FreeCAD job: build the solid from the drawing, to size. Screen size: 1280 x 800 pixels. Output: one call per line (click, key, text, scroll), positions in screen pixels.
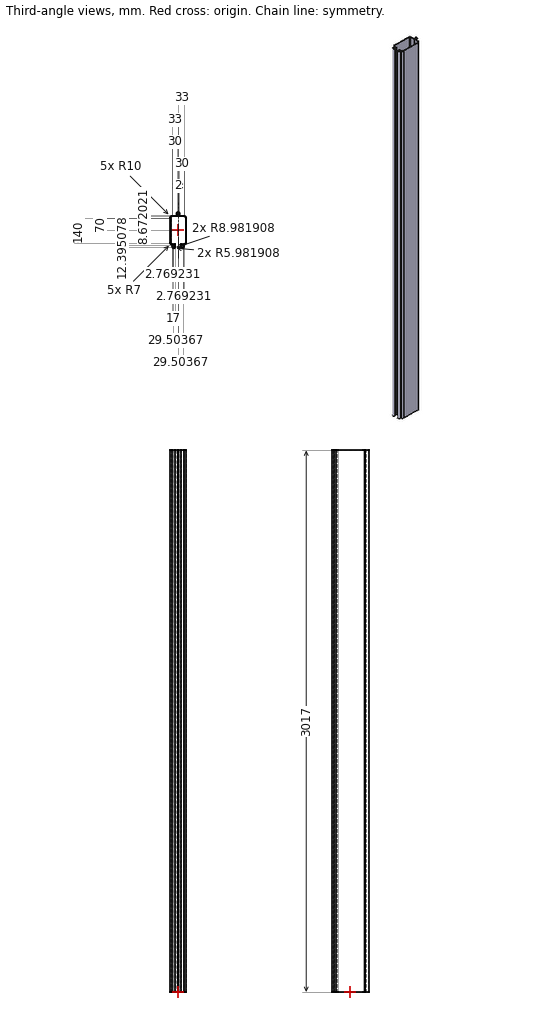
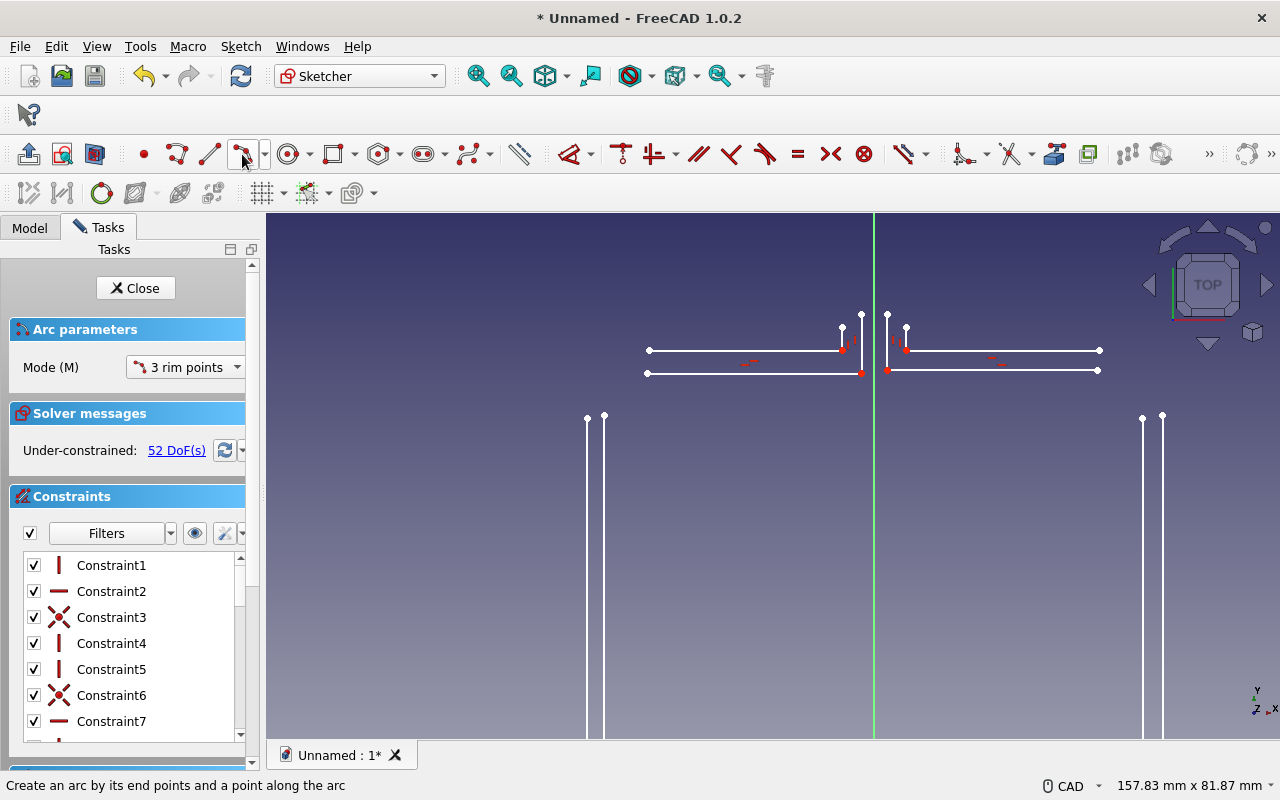
scroll(649, 350, down, 7)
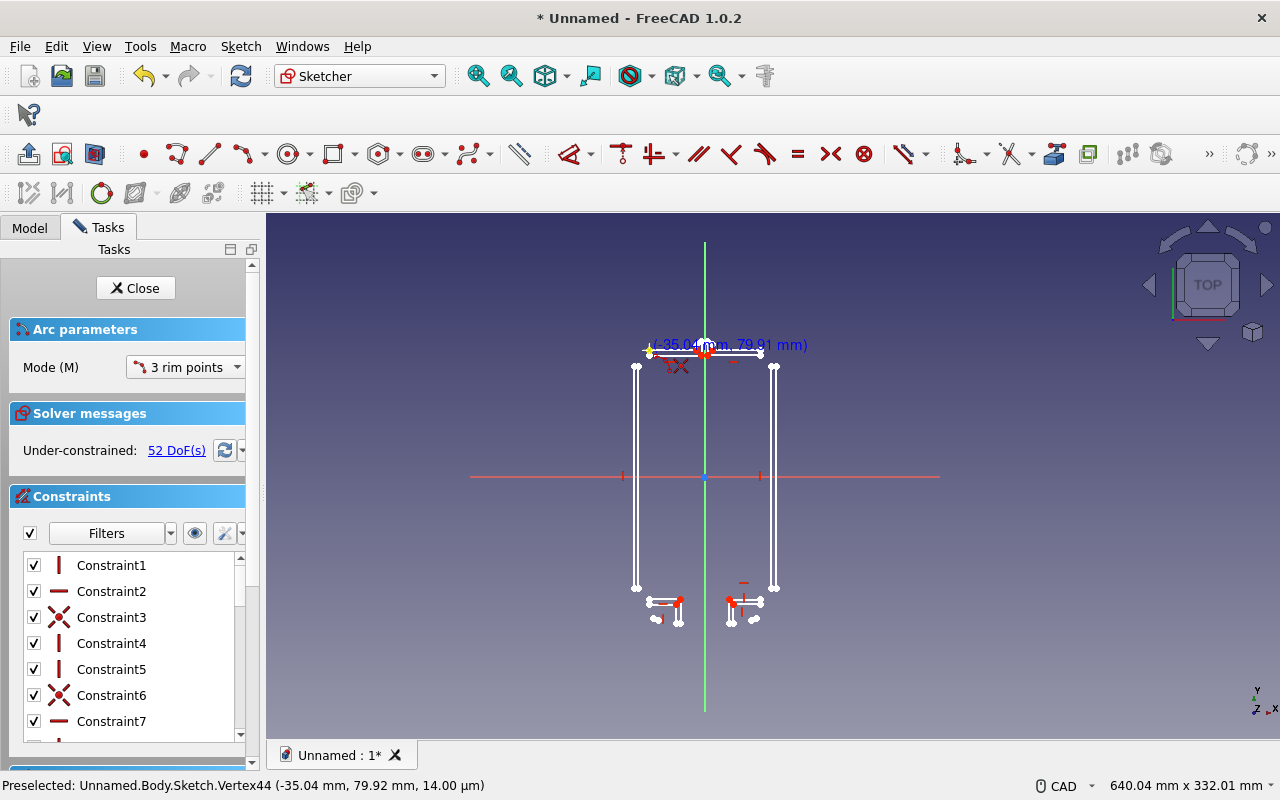
scroll(634, 588, up, 7)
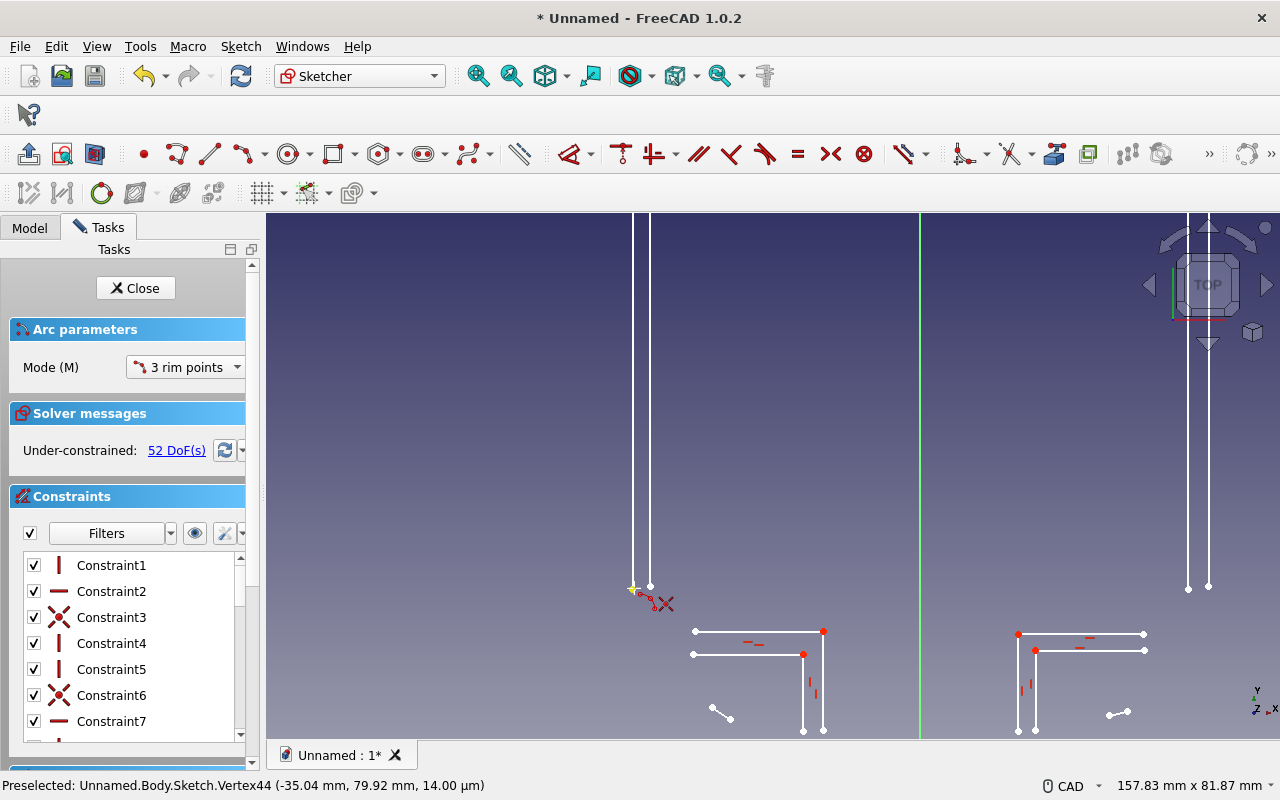
click(633, 590)
click(694, 655)
click(650, 631)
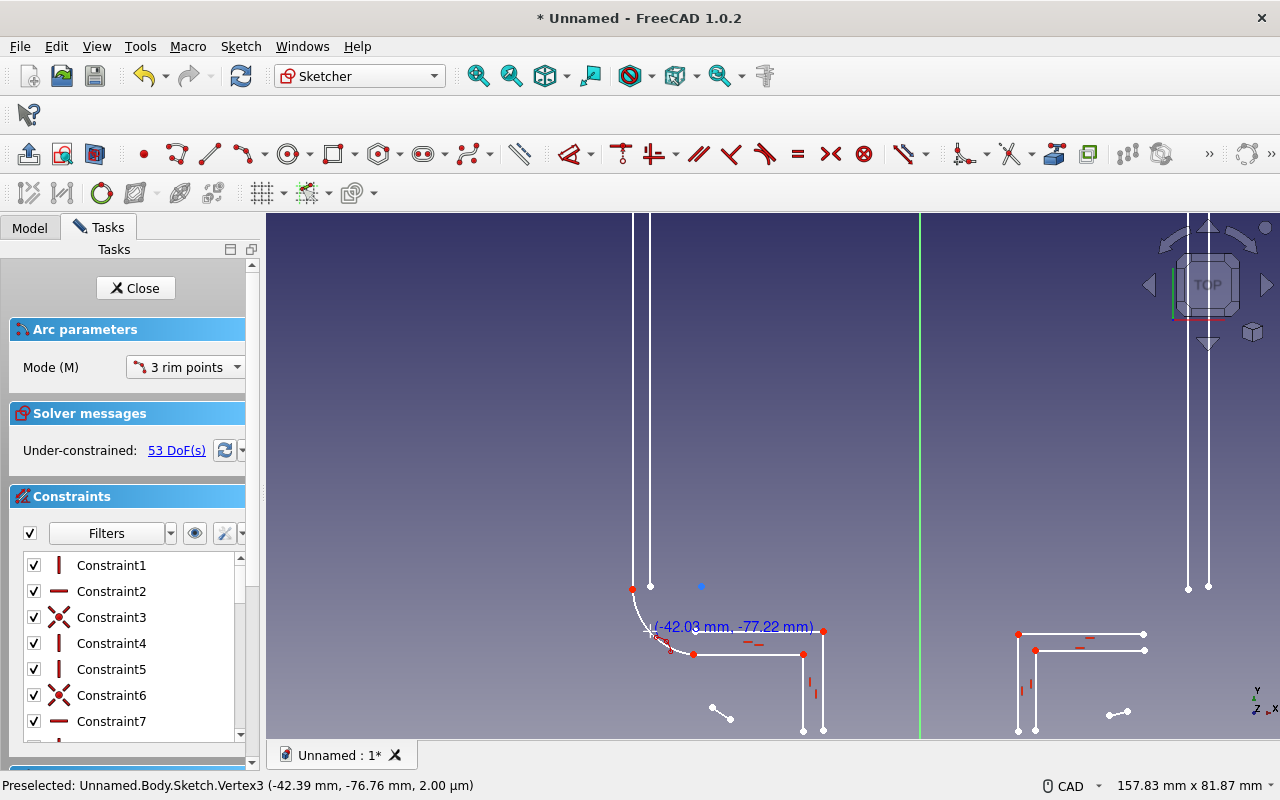
scroll(634, 589, down, 7)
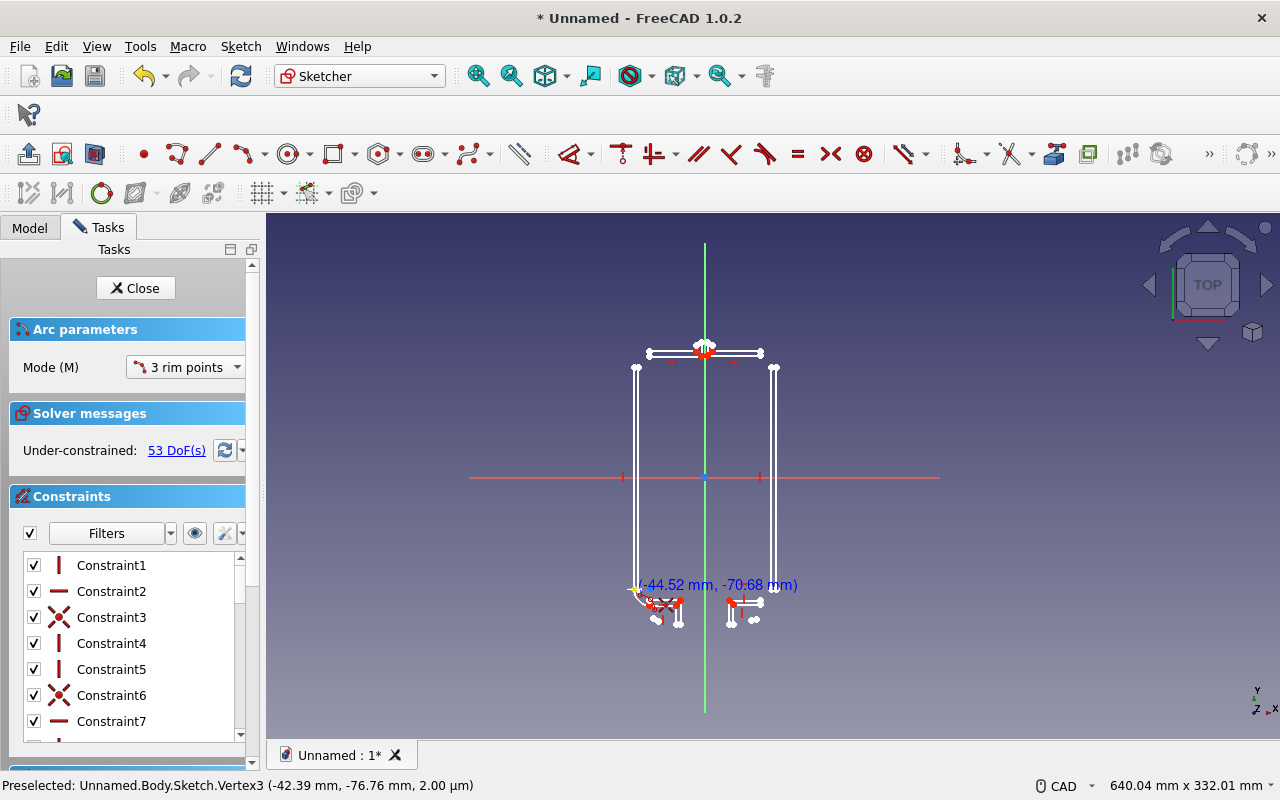
scroll(676, 624, up, 7)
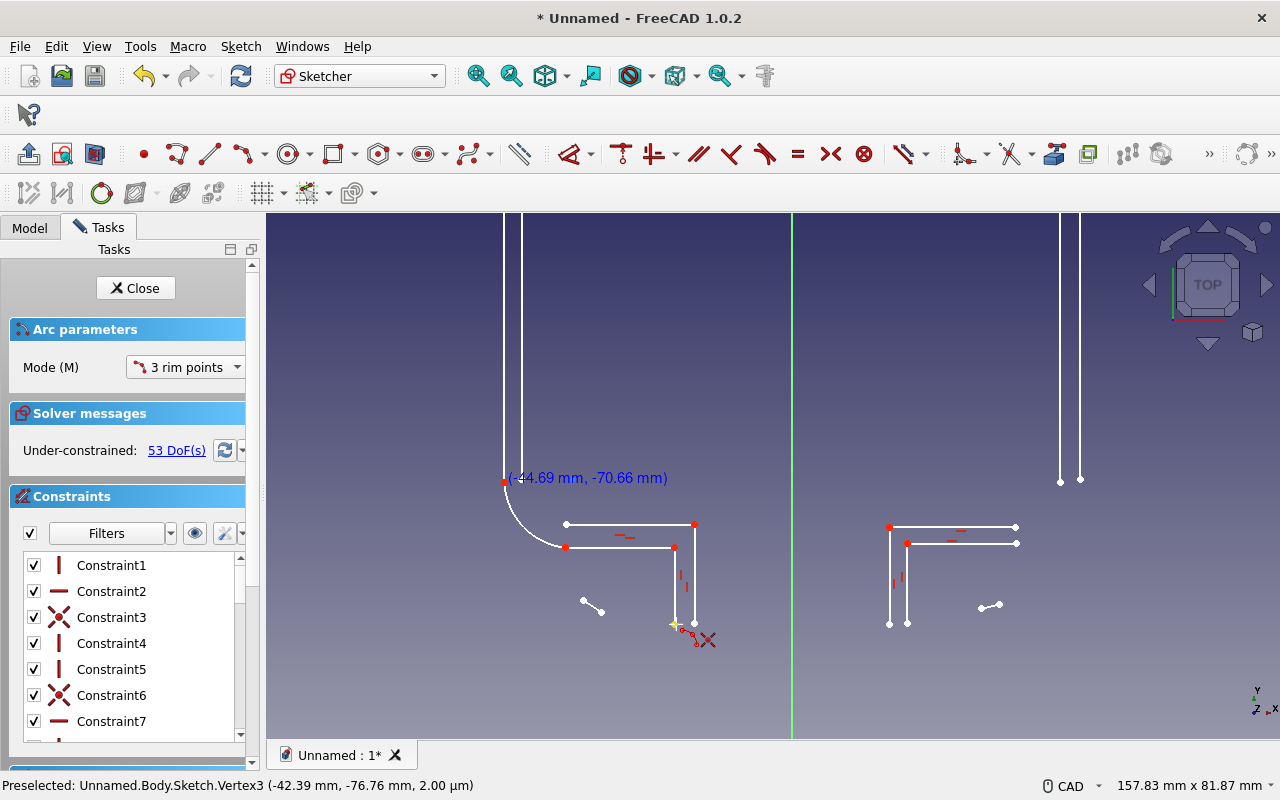
click(675, 625)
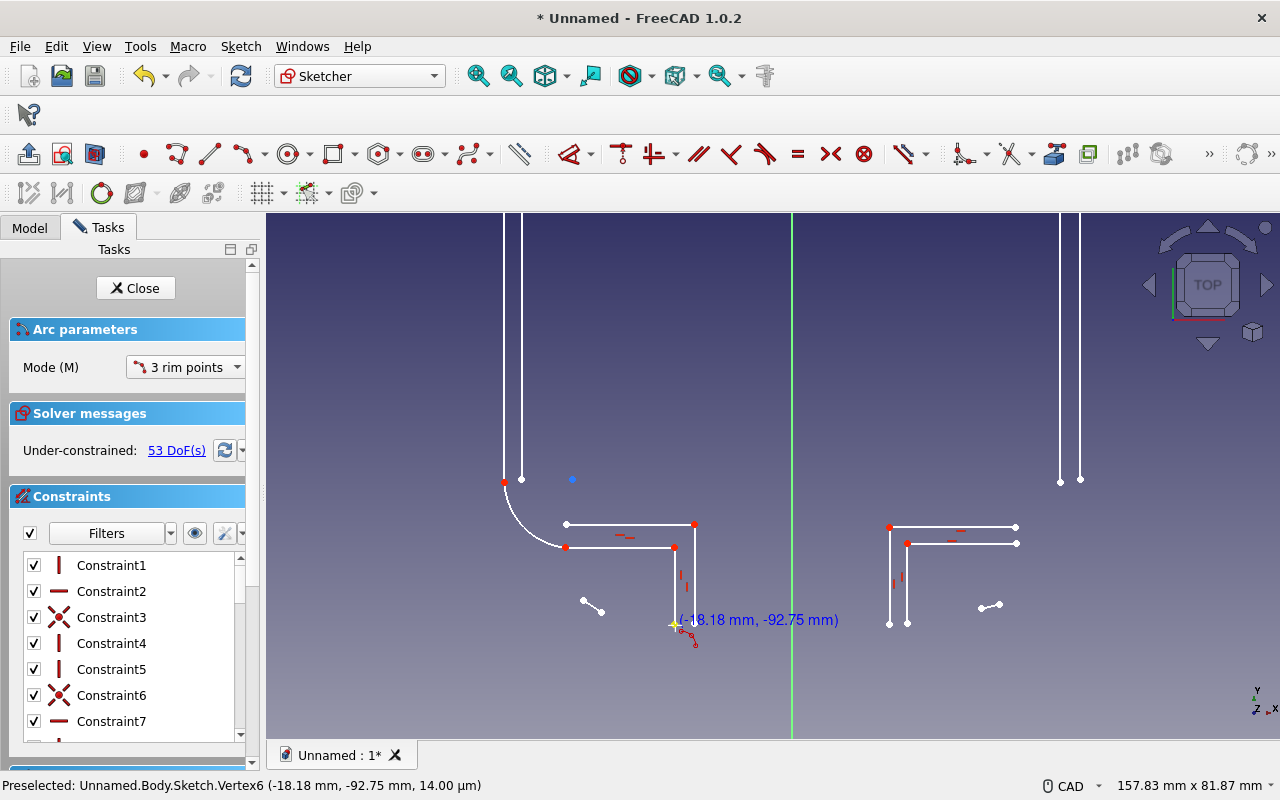
scroll(602, 608, up, 3)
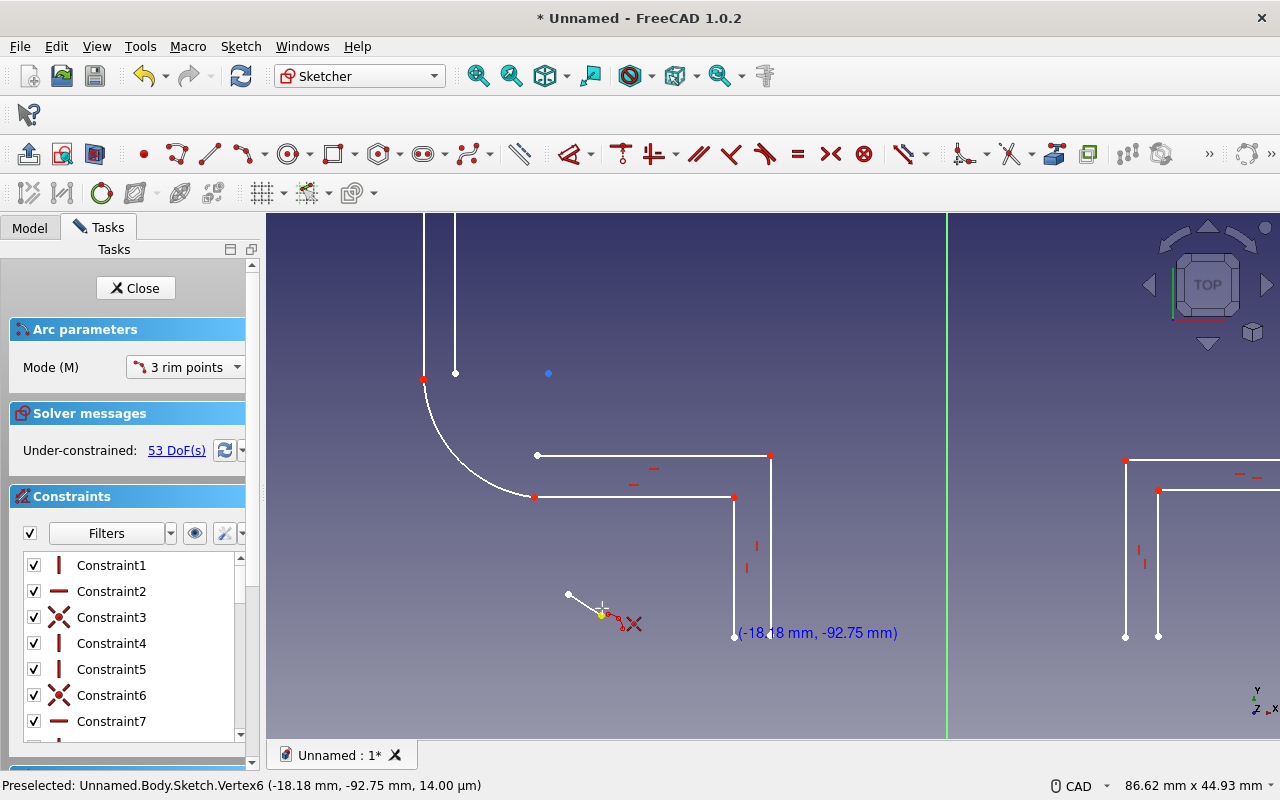
click(601, 616)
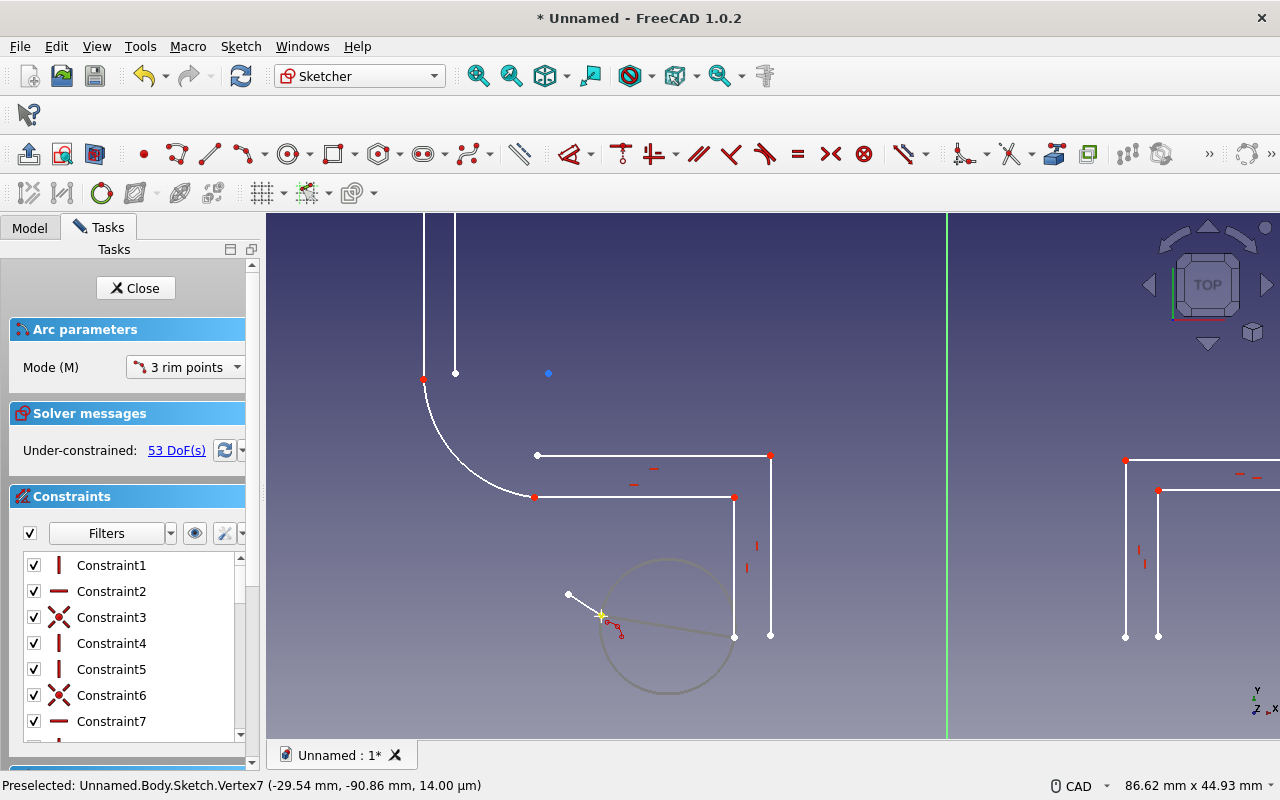
scroll(667, 622, down, 10)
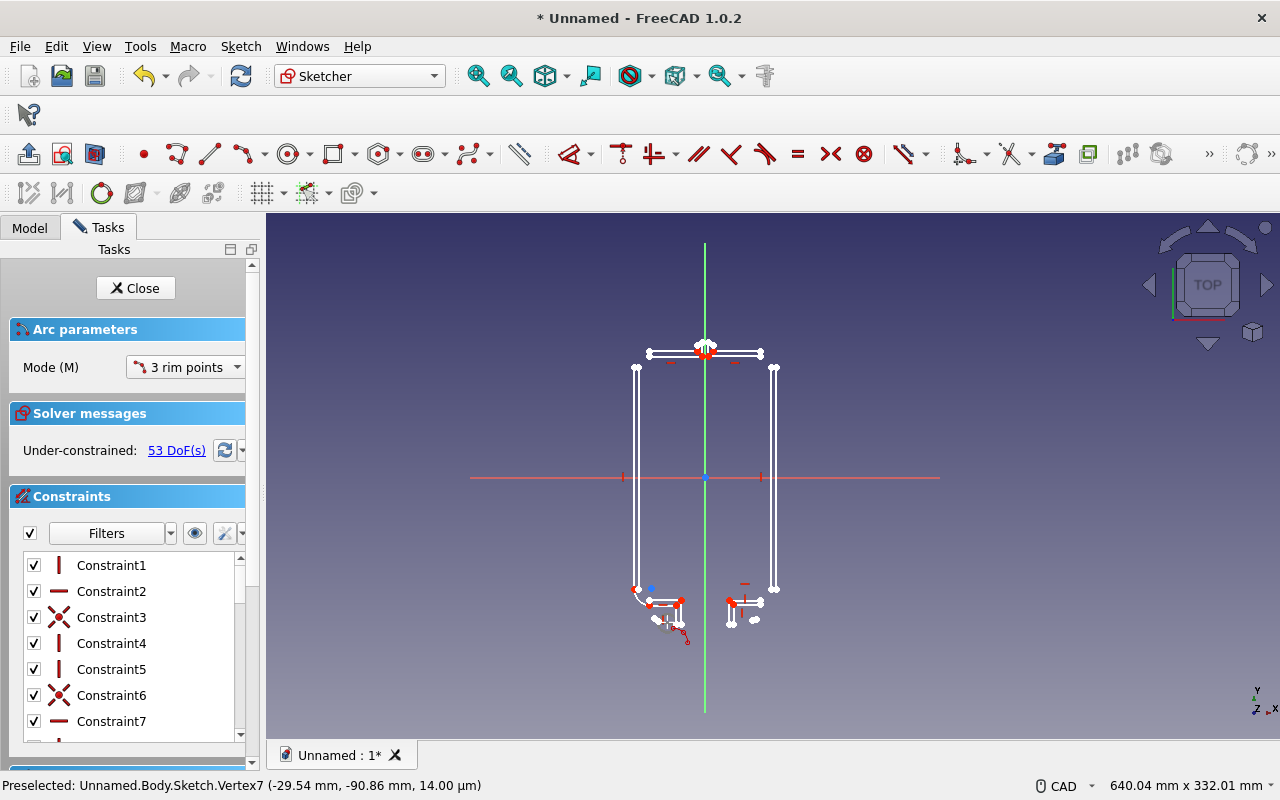
scroll(665, 634, up, 2)